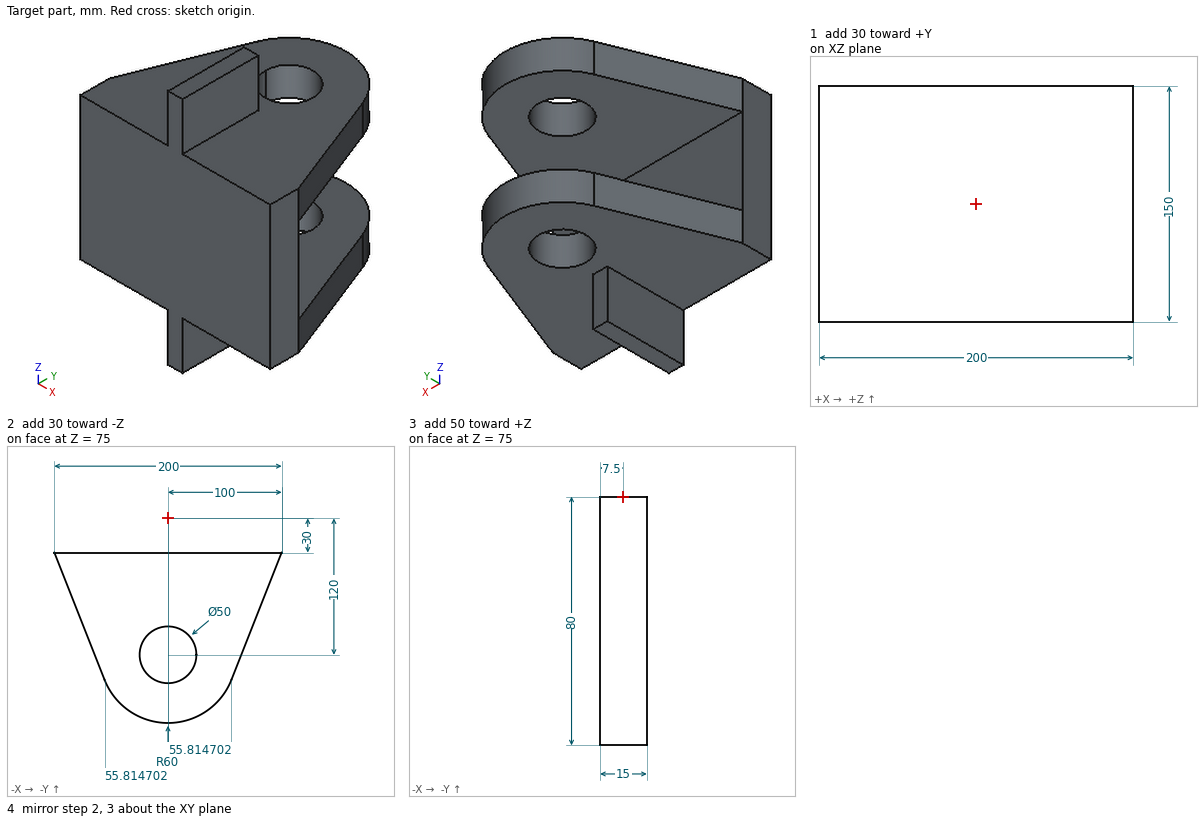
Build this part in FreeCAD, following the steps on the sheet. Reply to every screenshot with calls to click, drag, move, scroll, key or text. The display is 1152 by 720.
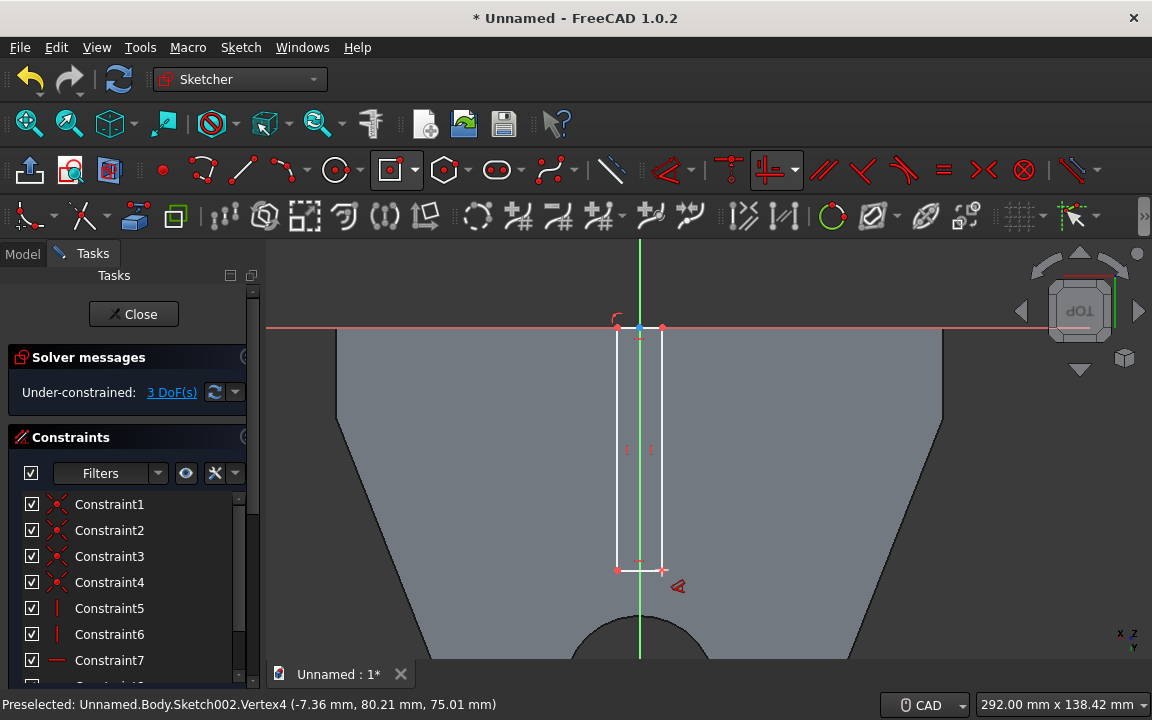
click(617, 401)
click(583, 449)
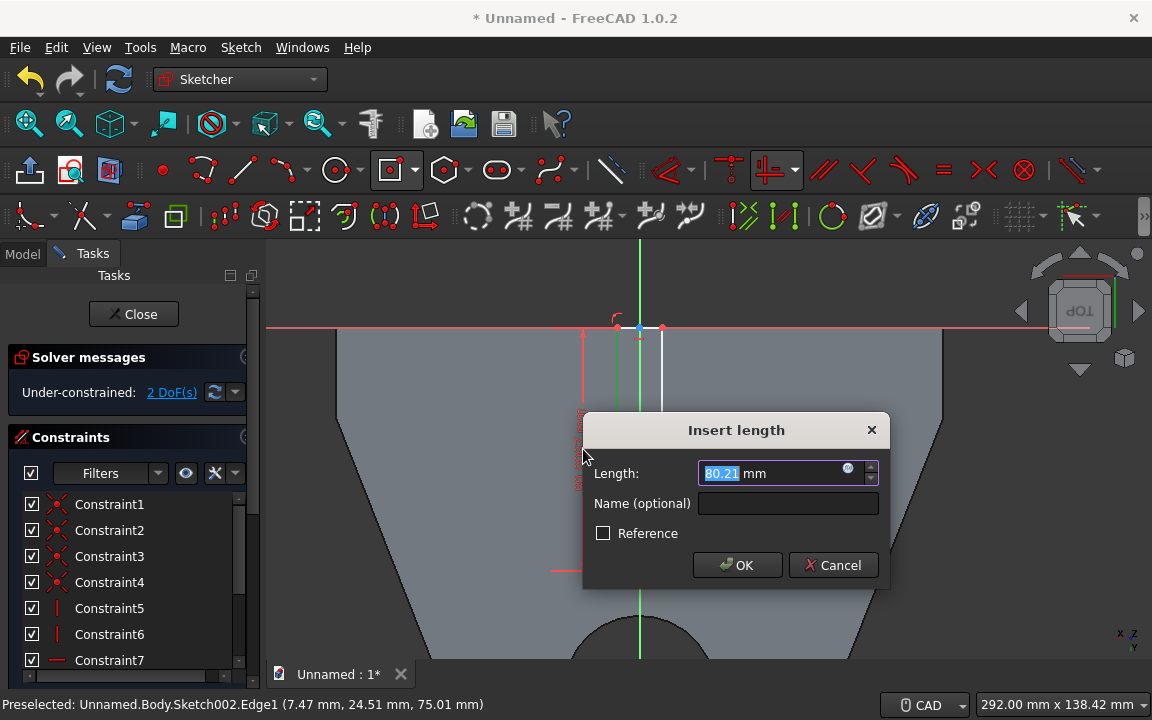
text(80)
key(Return)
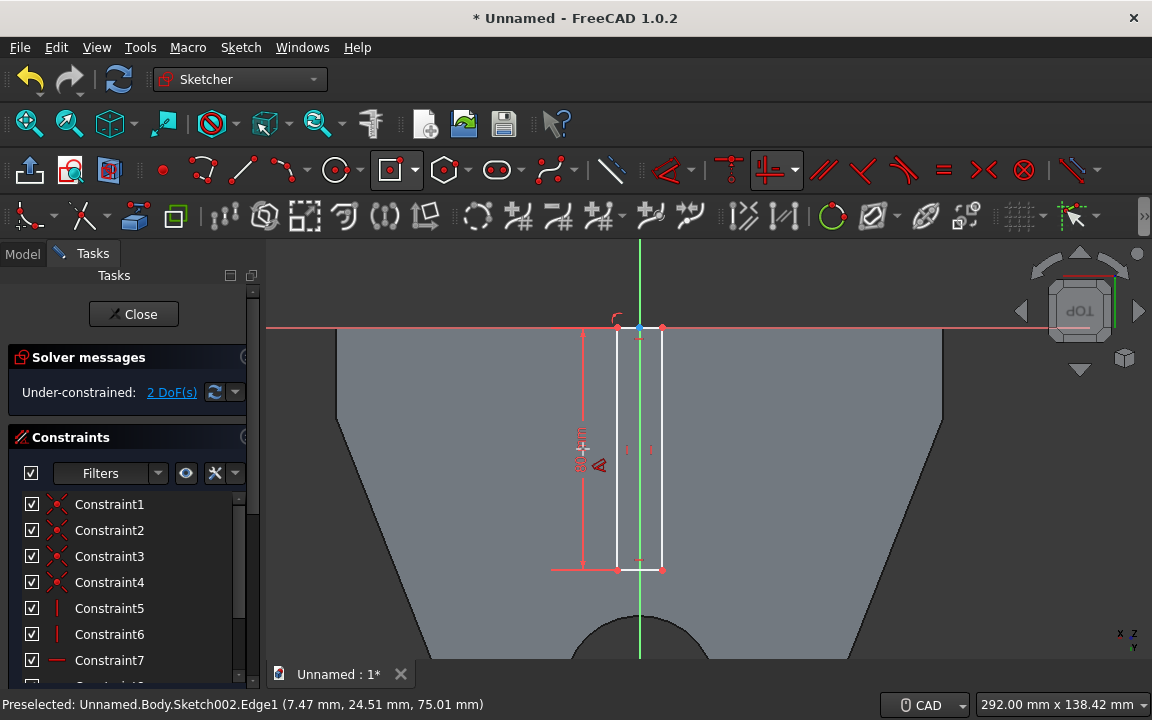
scroll(630, 570, up, 3)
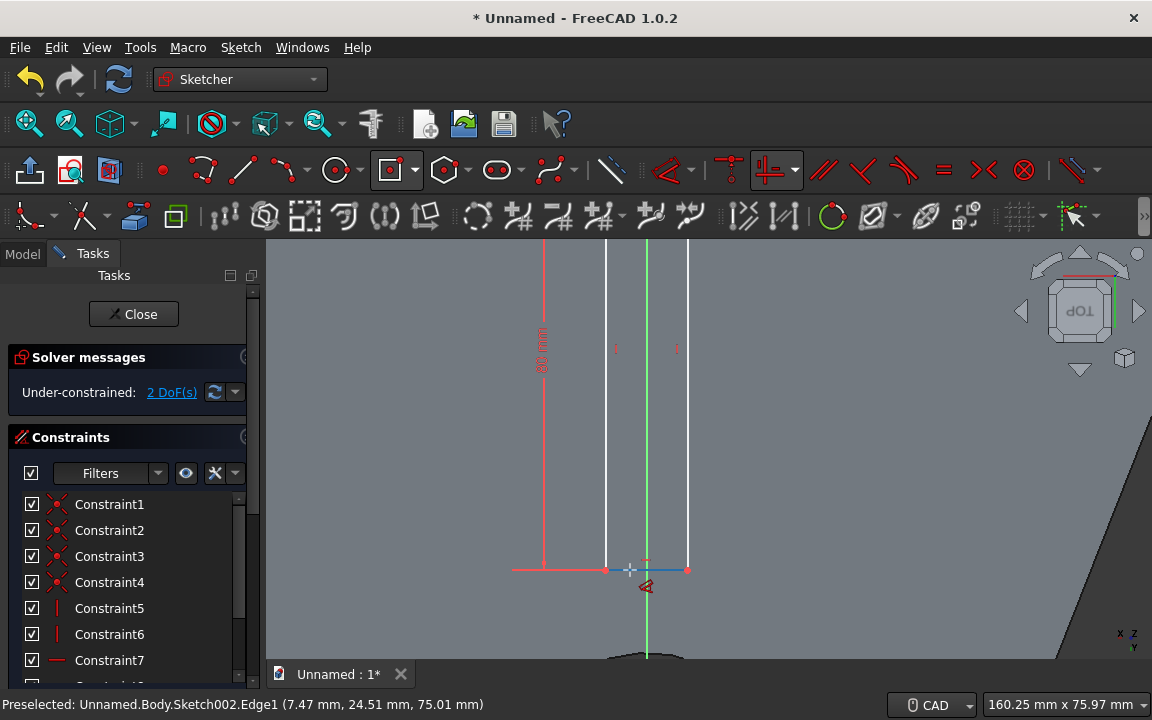
click(631, 570)
click(628, 604)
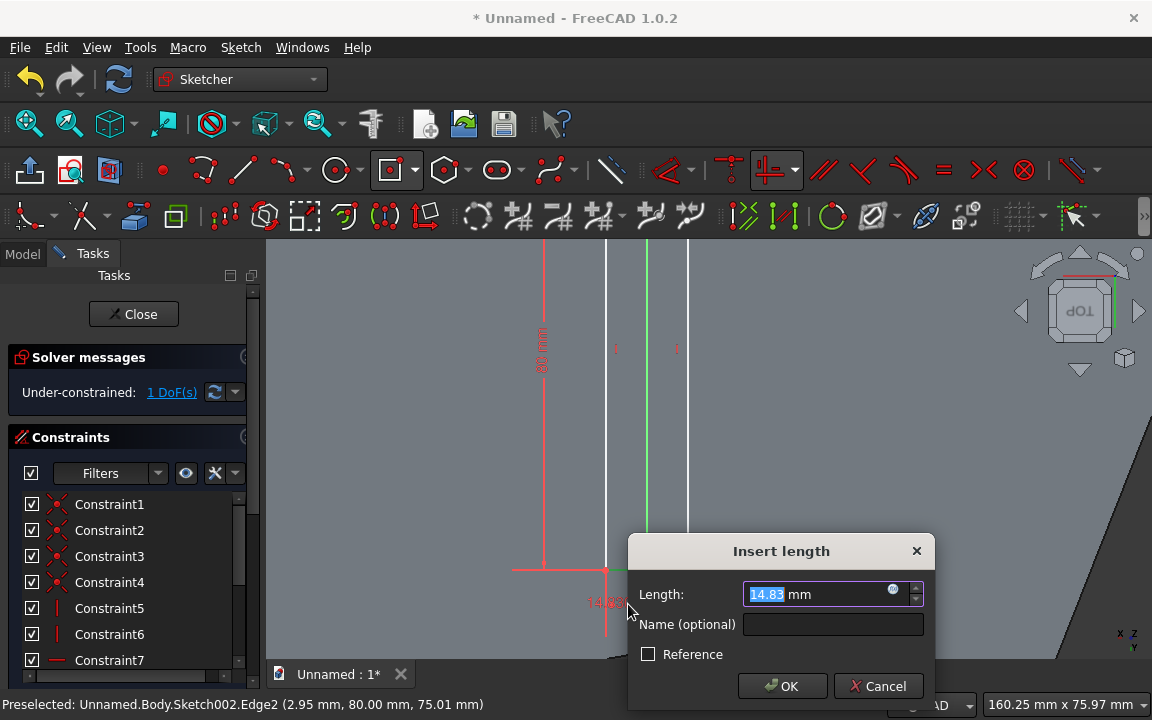
text(15)
key(Return)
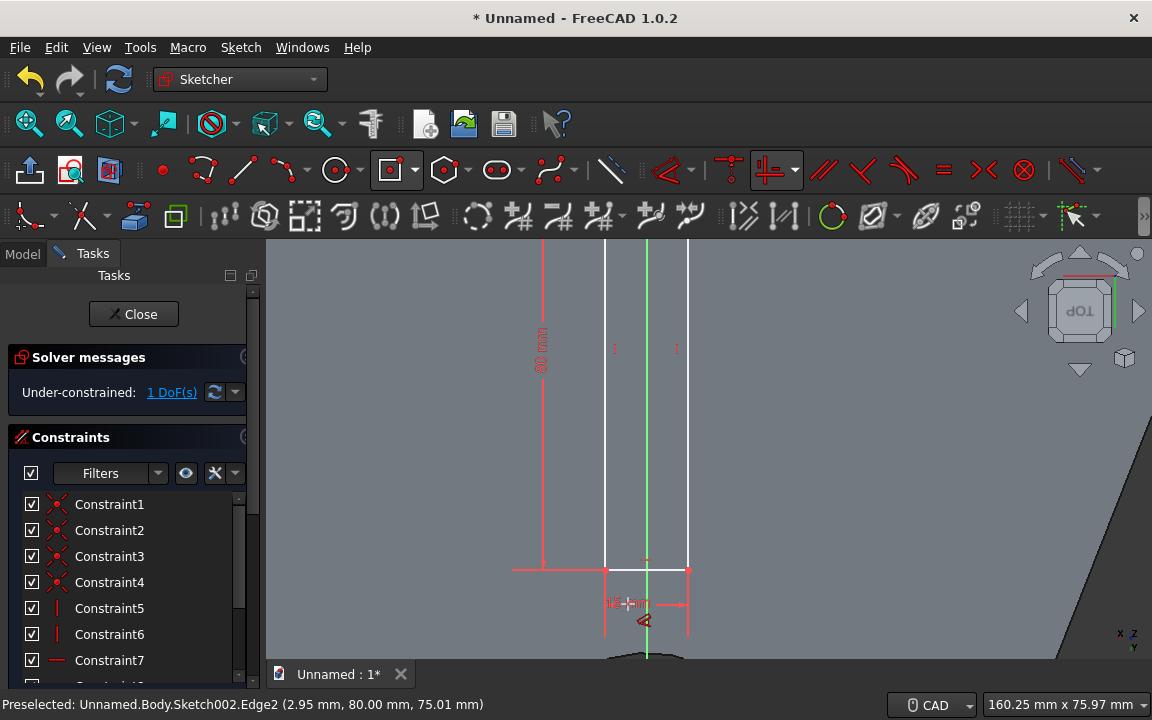
scroll(632, 571, down, 3)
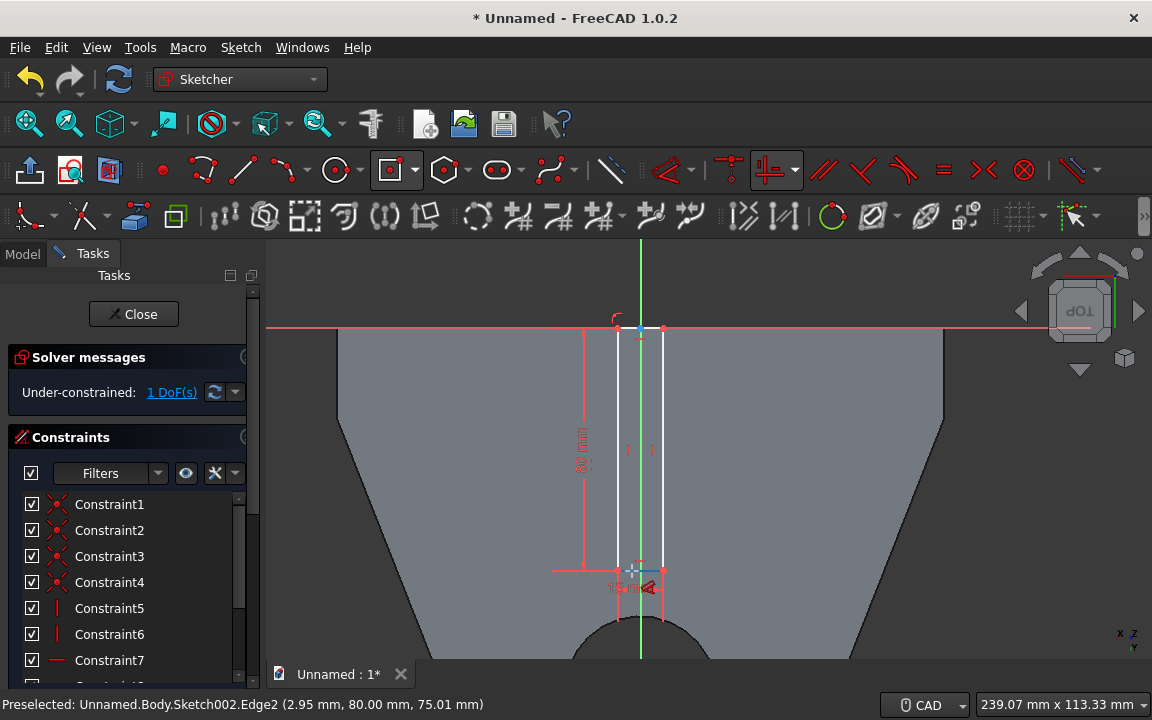
scroll(618, 328, up, 3)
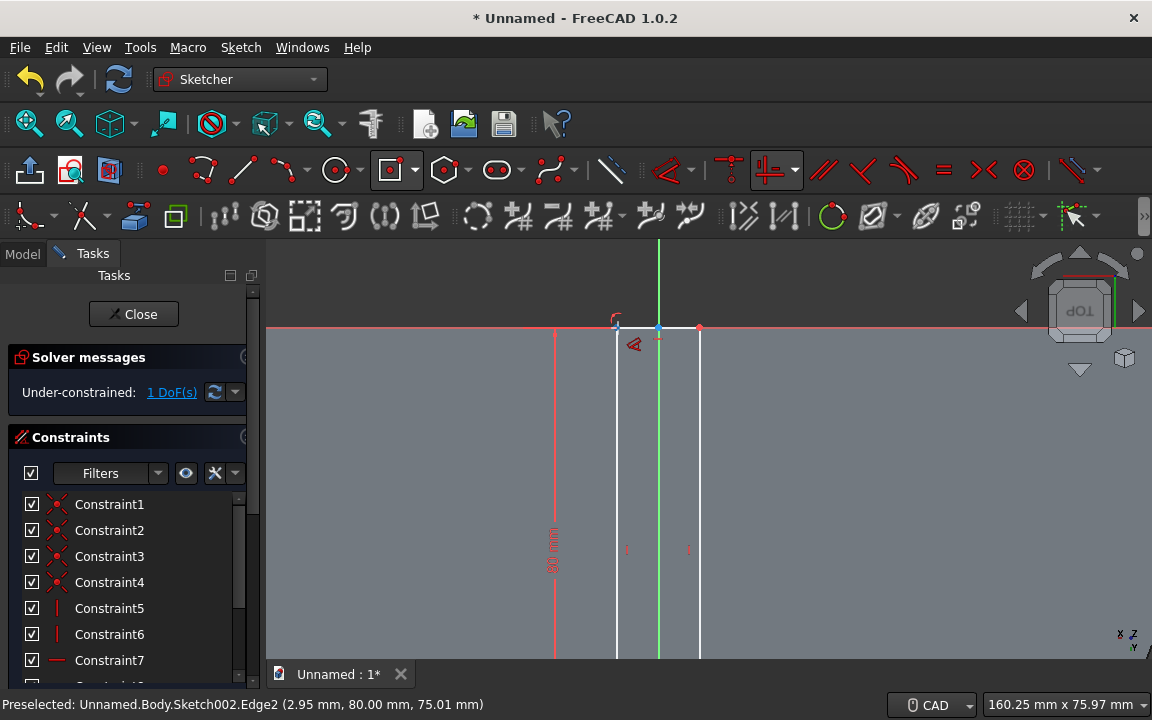
click(617, 328)
click(638, 294)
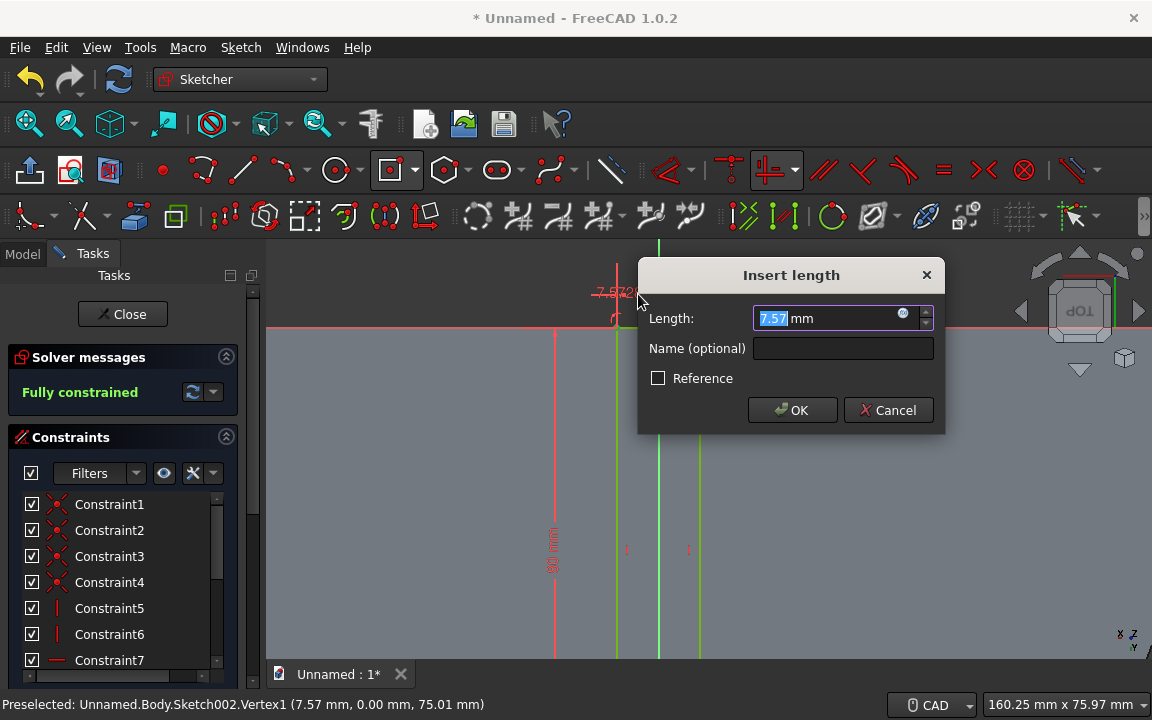
text(7.5)
key(Return)
key(Escape)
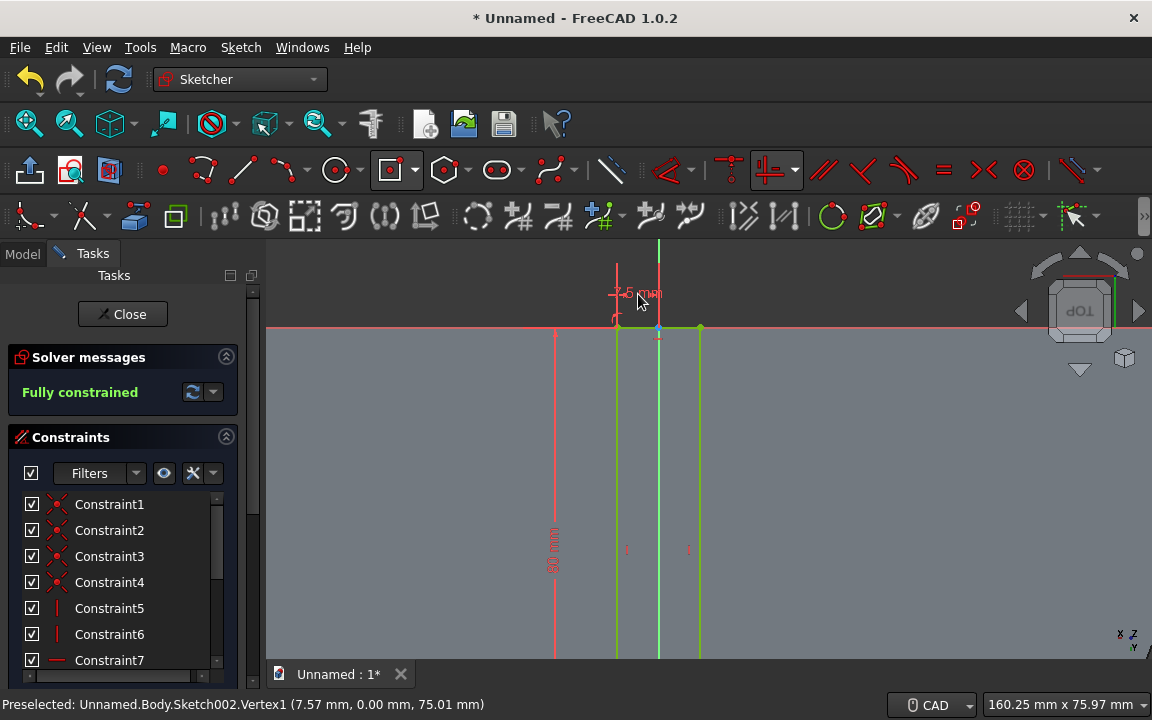
click(123, 314)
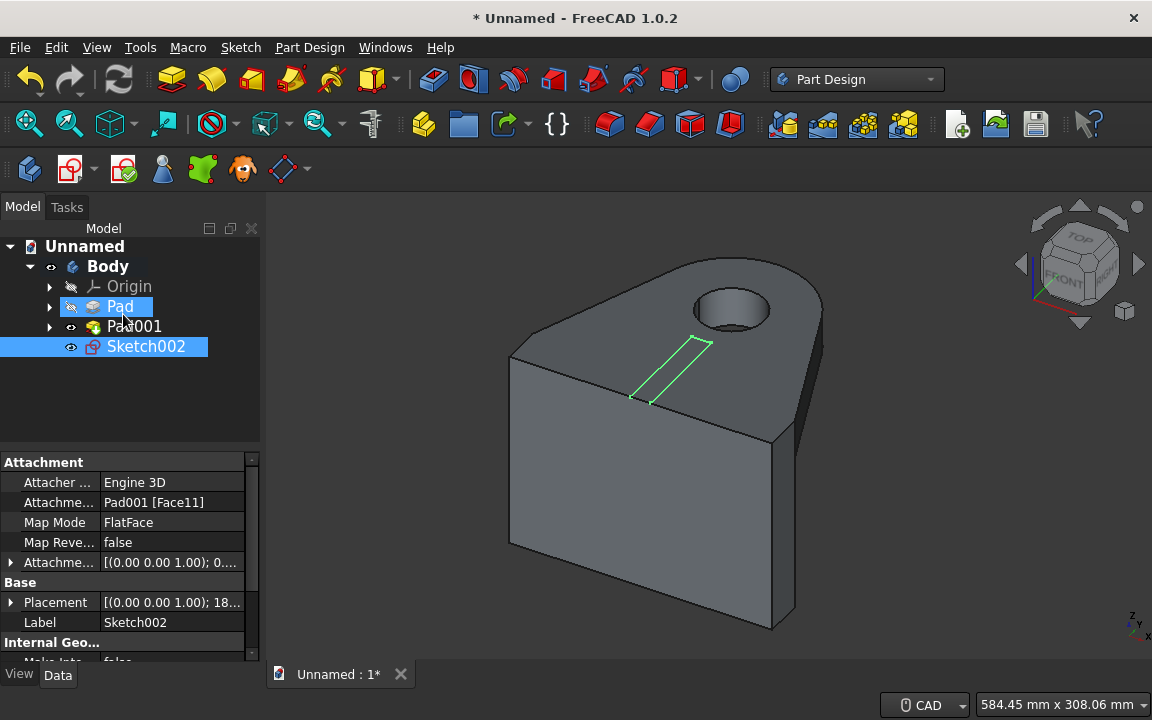
click(172, 80)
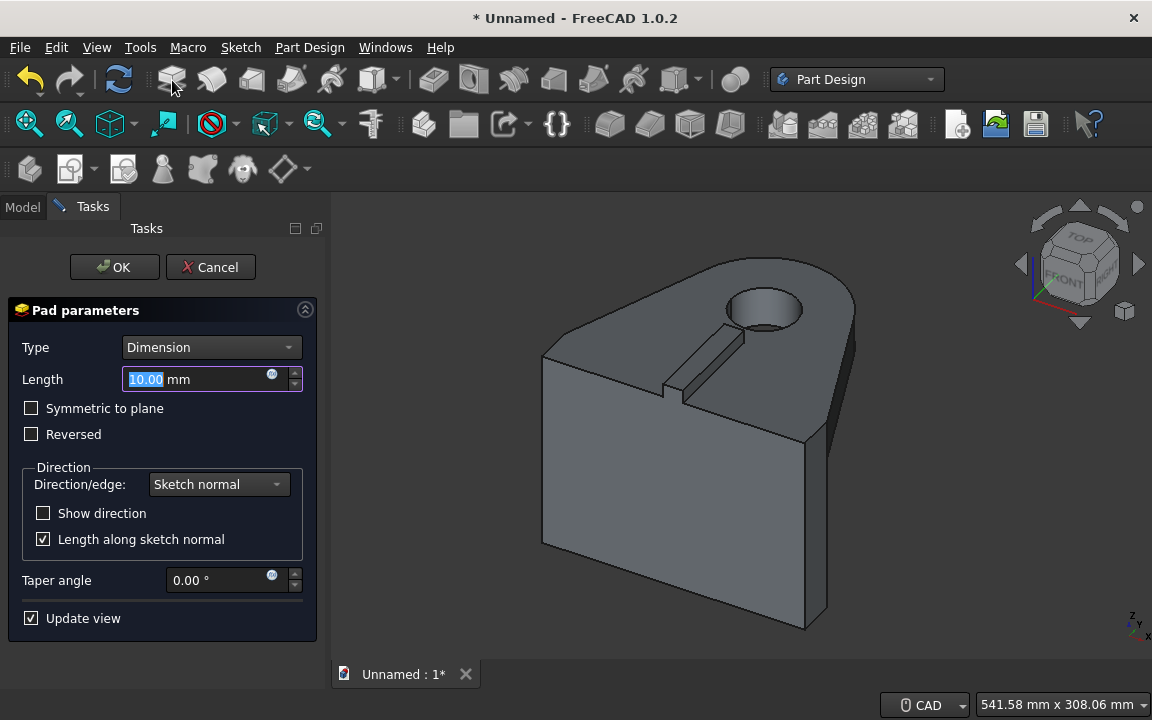
text(50)
key(Tab)